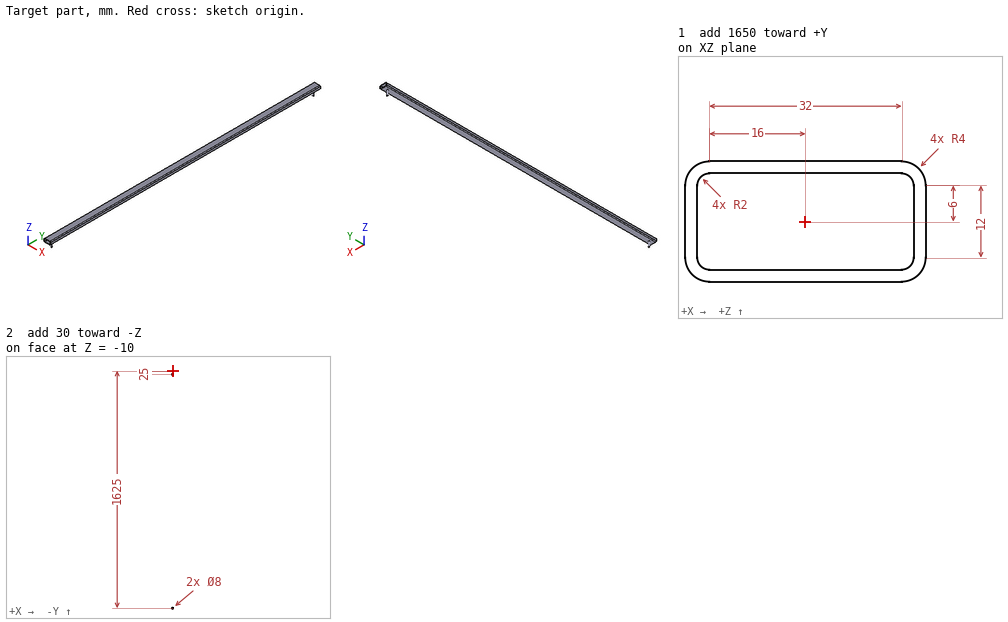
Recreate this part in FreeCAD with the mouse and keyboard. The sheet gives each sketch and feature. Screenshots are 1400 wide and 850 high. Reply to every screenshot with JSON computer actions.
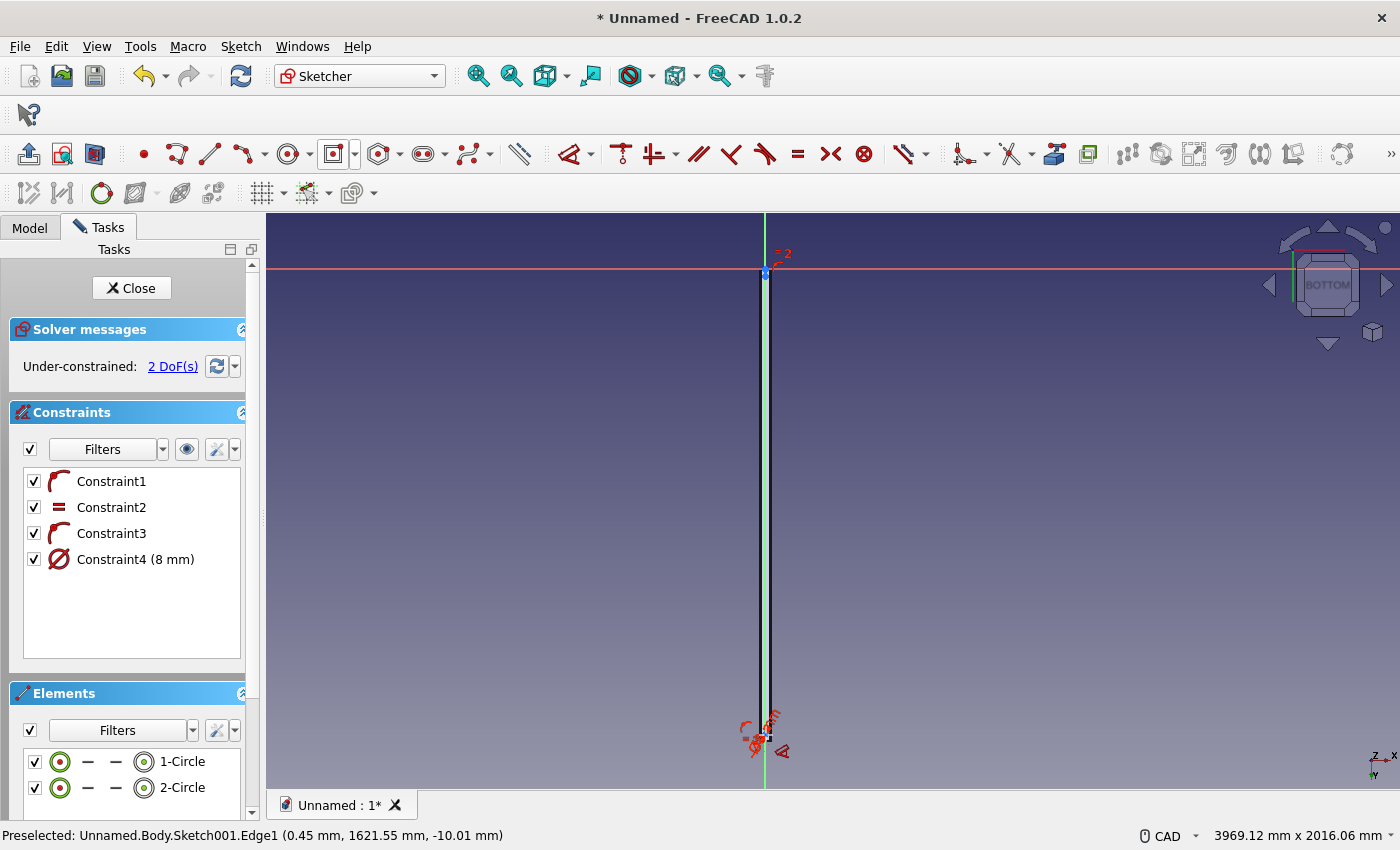
{"action": "scroll", "coordinate": [765, 277], "scroll_direction": "up", "scroll_amount": 9}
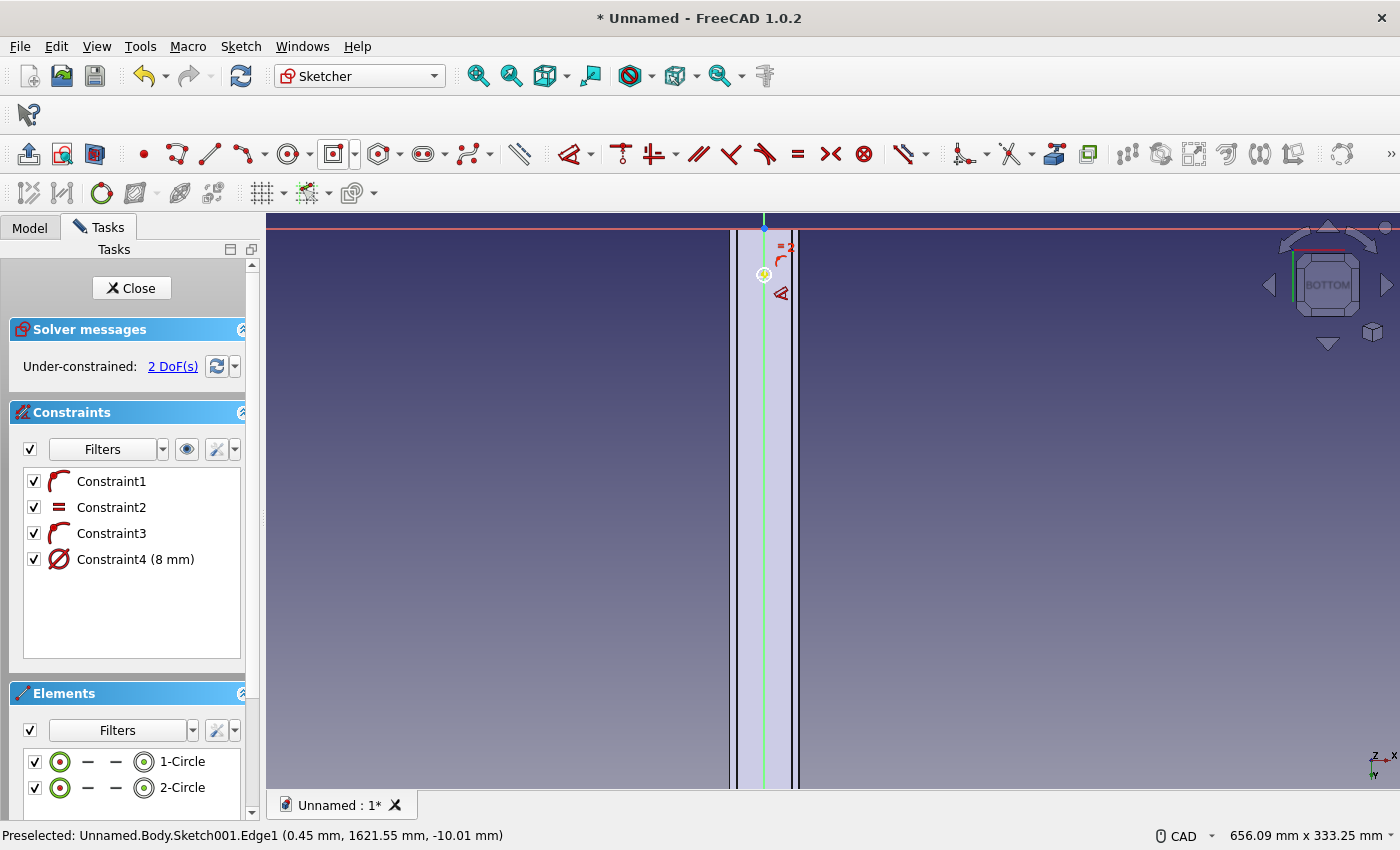
{"action": "left_click", "coordinate": [764, 275]}
{"action": "left_click", "coordinate": [798, 258]}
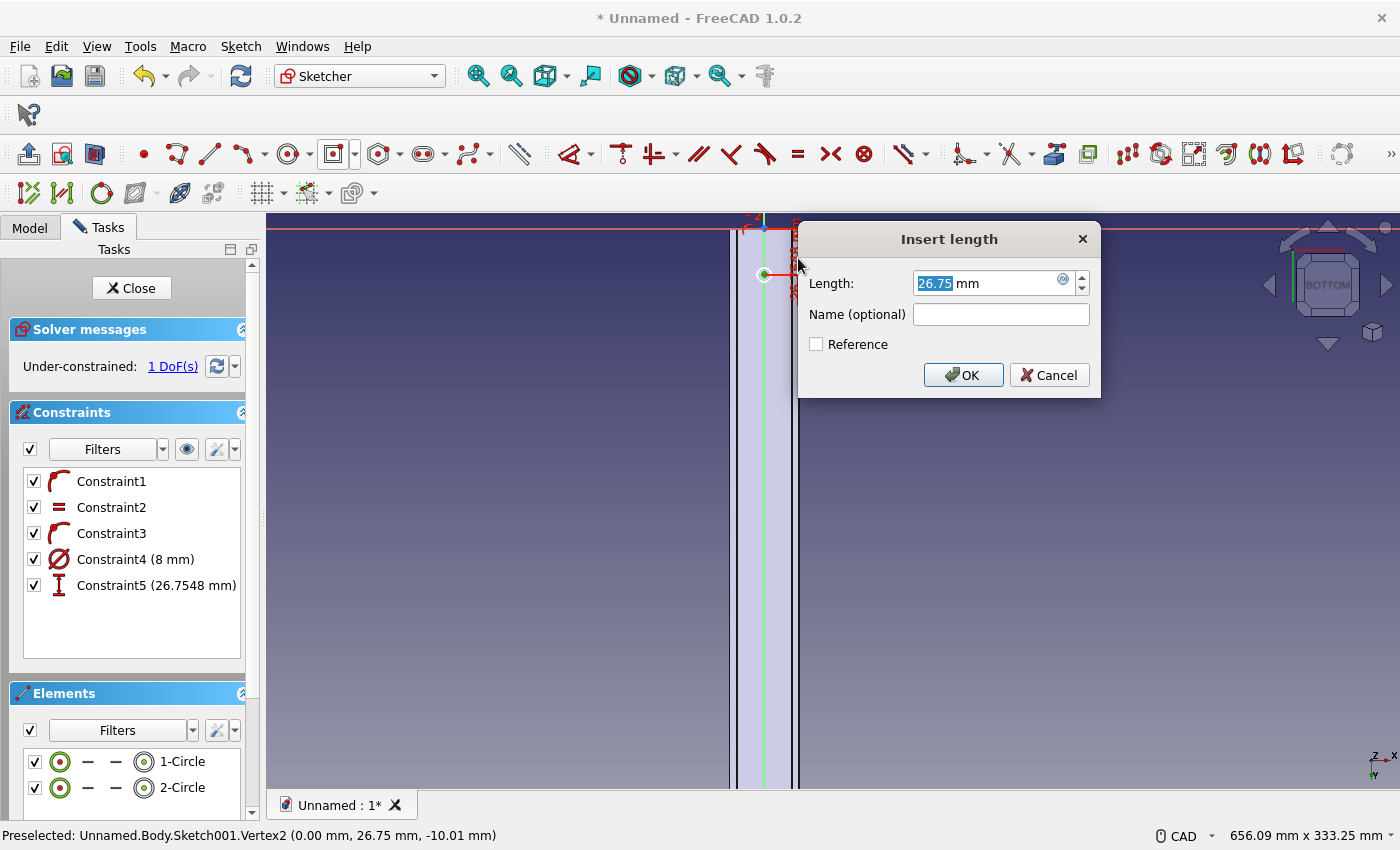
{"action": "type", "text": "25"}
{"action": "key", "text": "Return"}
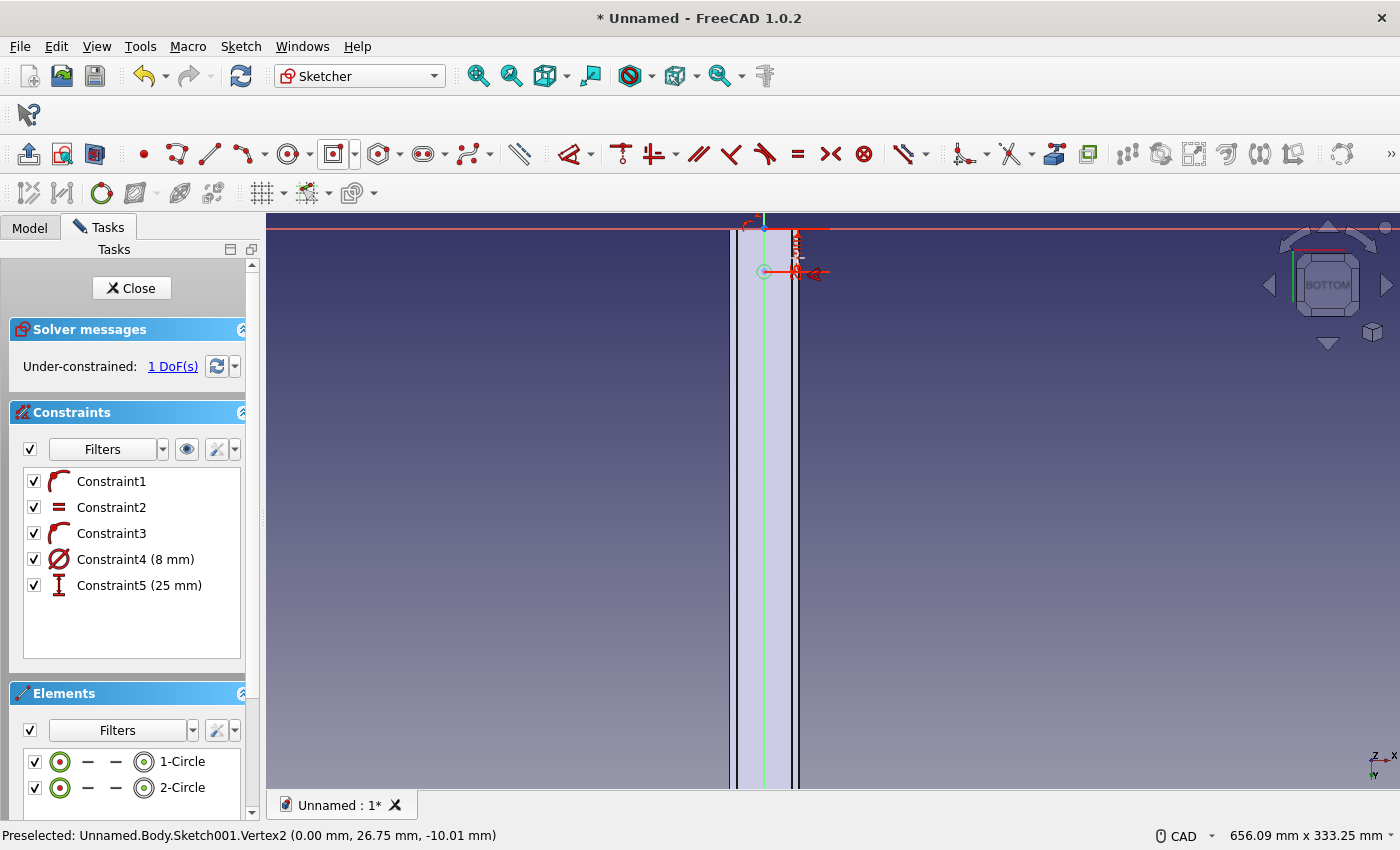
{"action": "scroll", "coordinate": [765, 323], "scroll_direction": "down", "scroll_amount": 10}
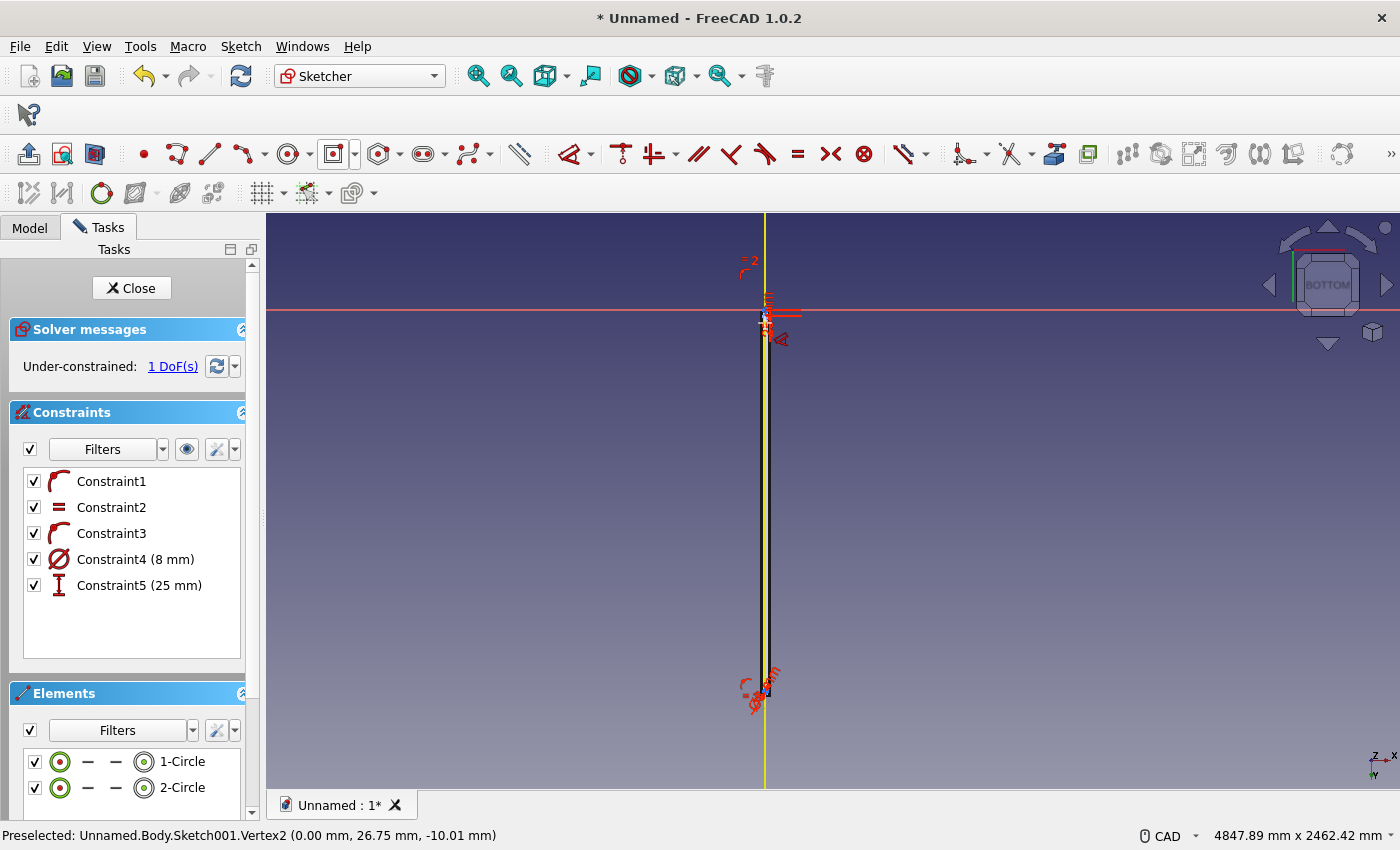
{"action": "left_click", "coordinate": [765, 691]}
{"action": "left_click", "coordinate": [799, 501]}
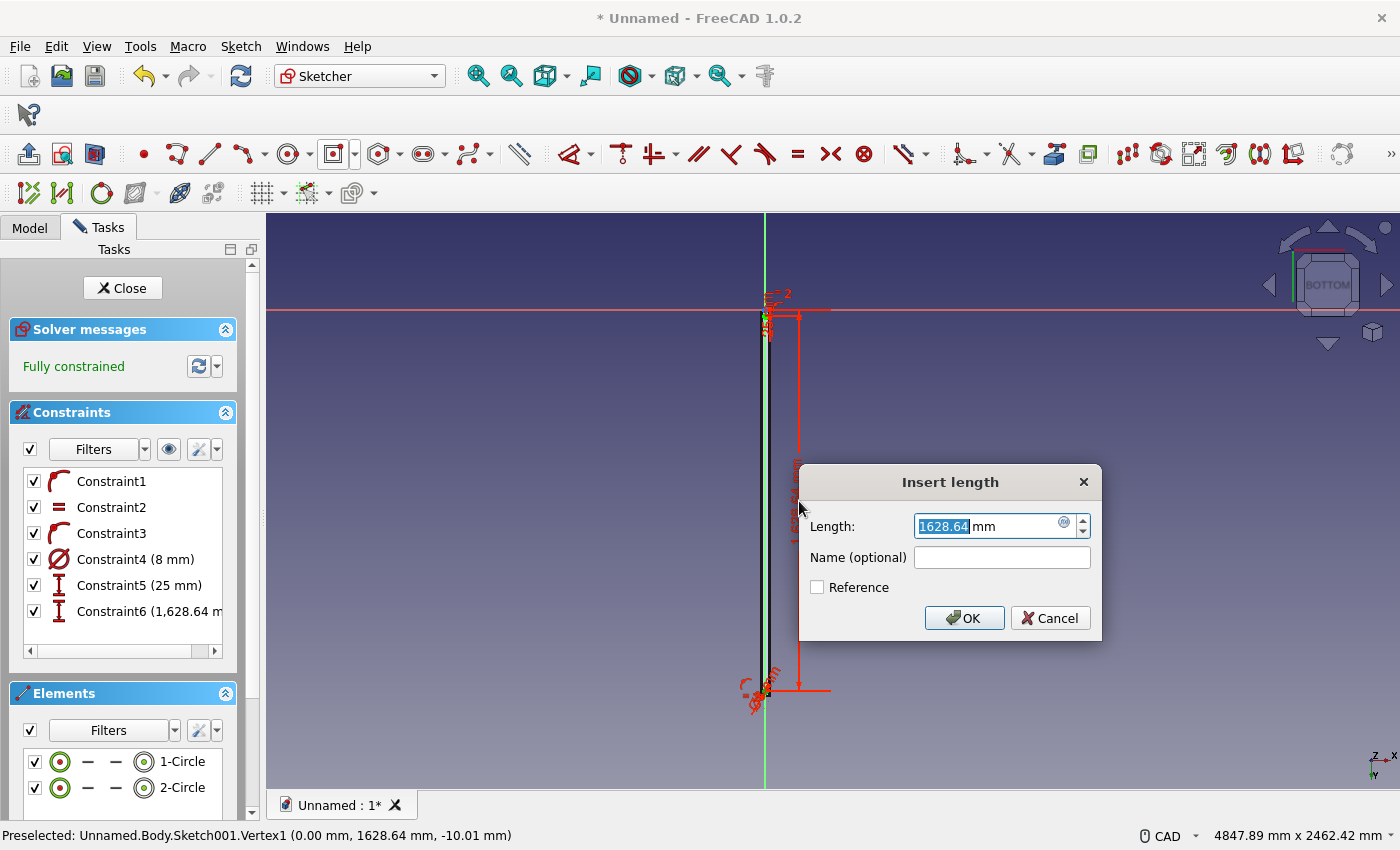
{"action": "type", "text": "1625"}
{"action": "key", "text": "Return"}
{"action": "key", "text": "Escape"}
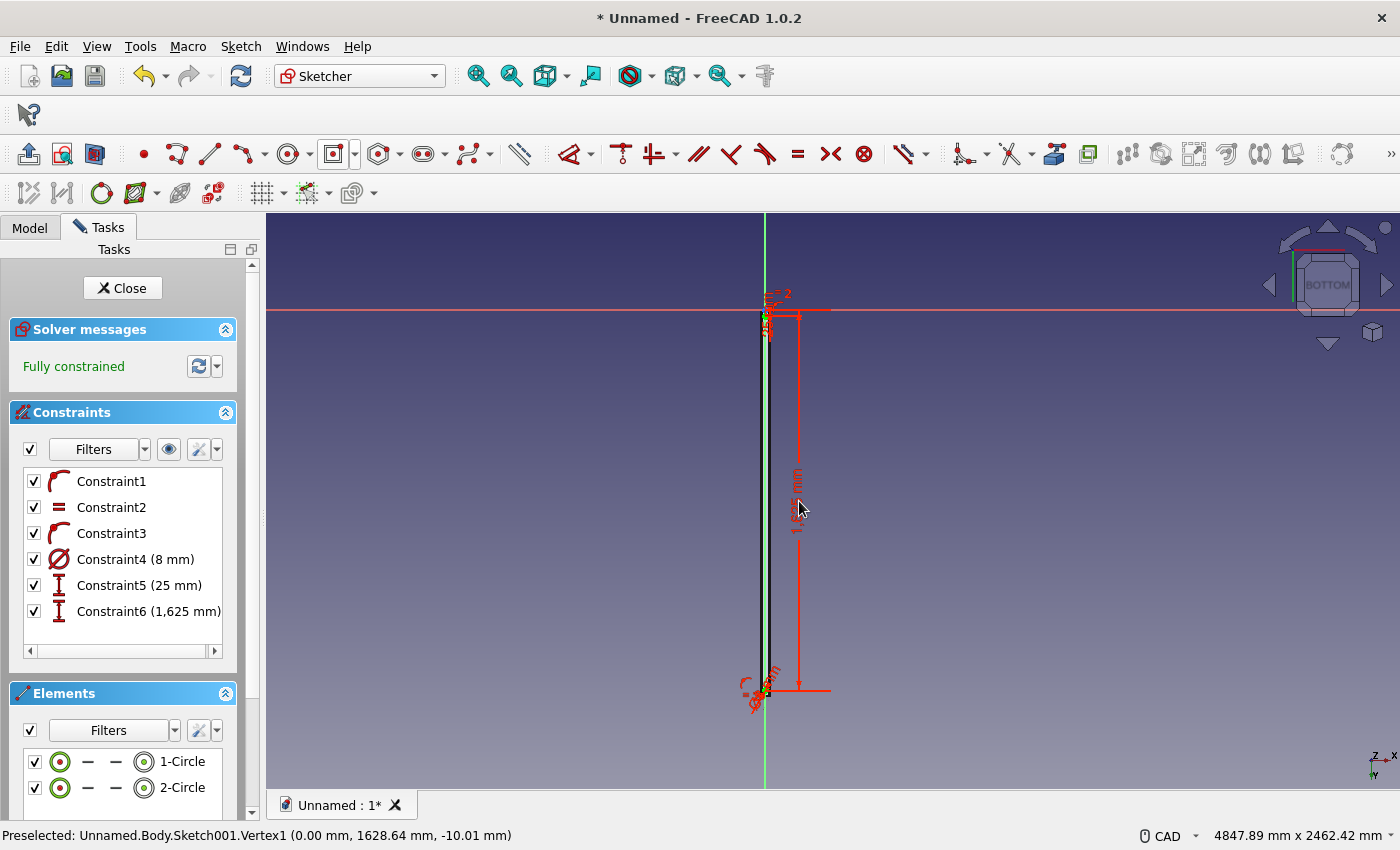
{"action": "left_click", "coordinate": [123, 288]}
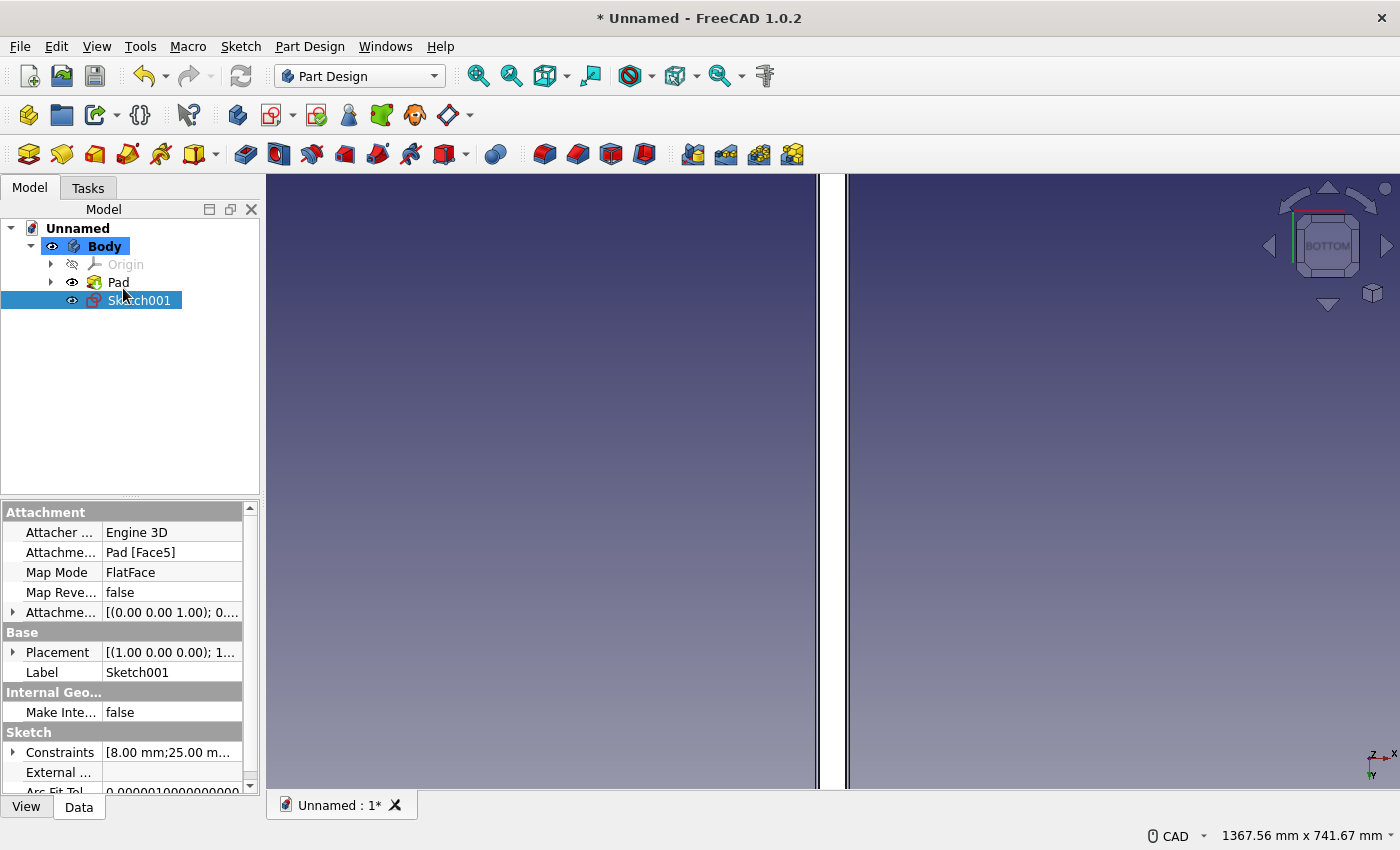
{"action": "left_click", "coordinate": [29, 154]}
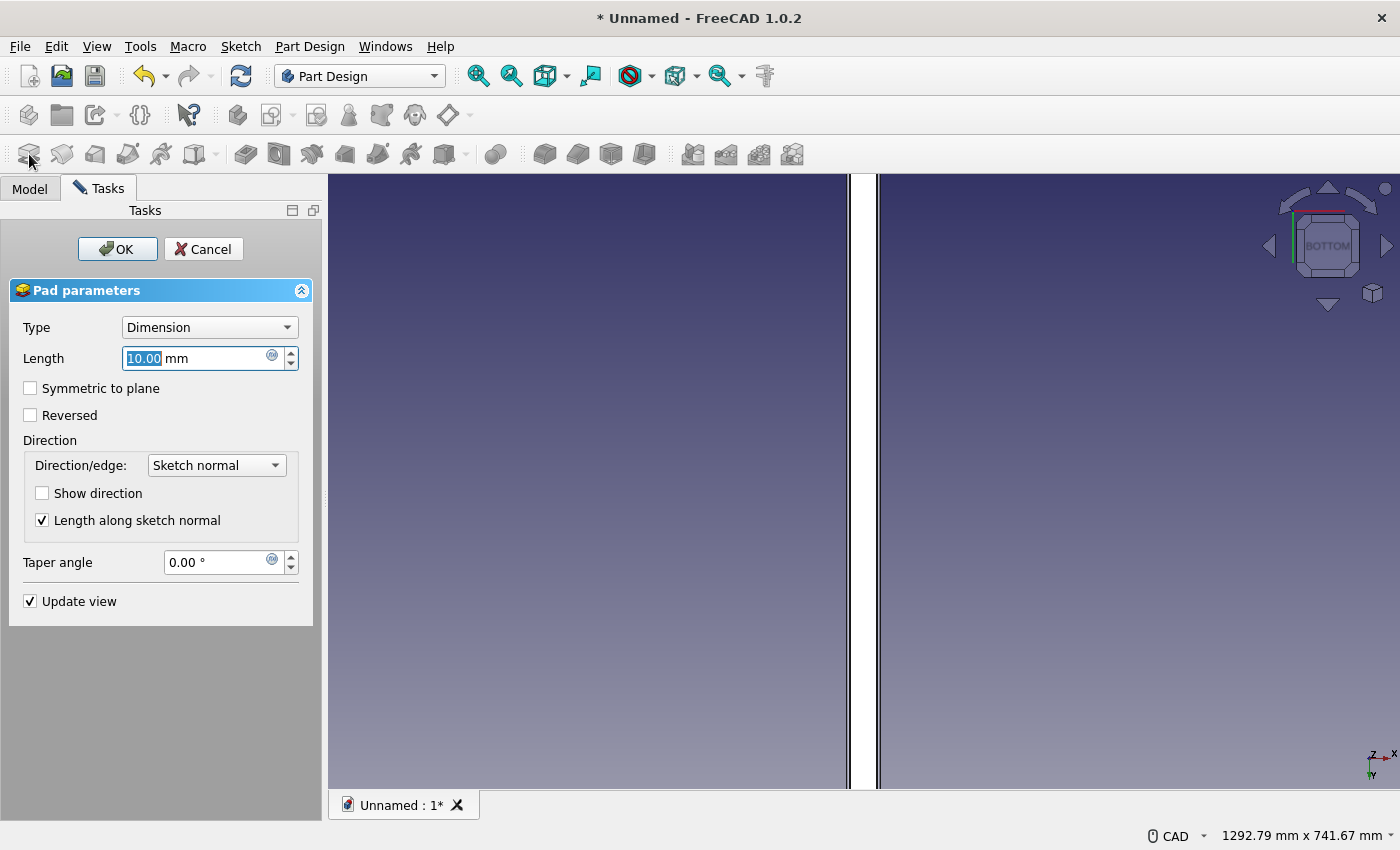
{"action": "type", "text": "30"}
{"action": "key", "text": "Tab"}